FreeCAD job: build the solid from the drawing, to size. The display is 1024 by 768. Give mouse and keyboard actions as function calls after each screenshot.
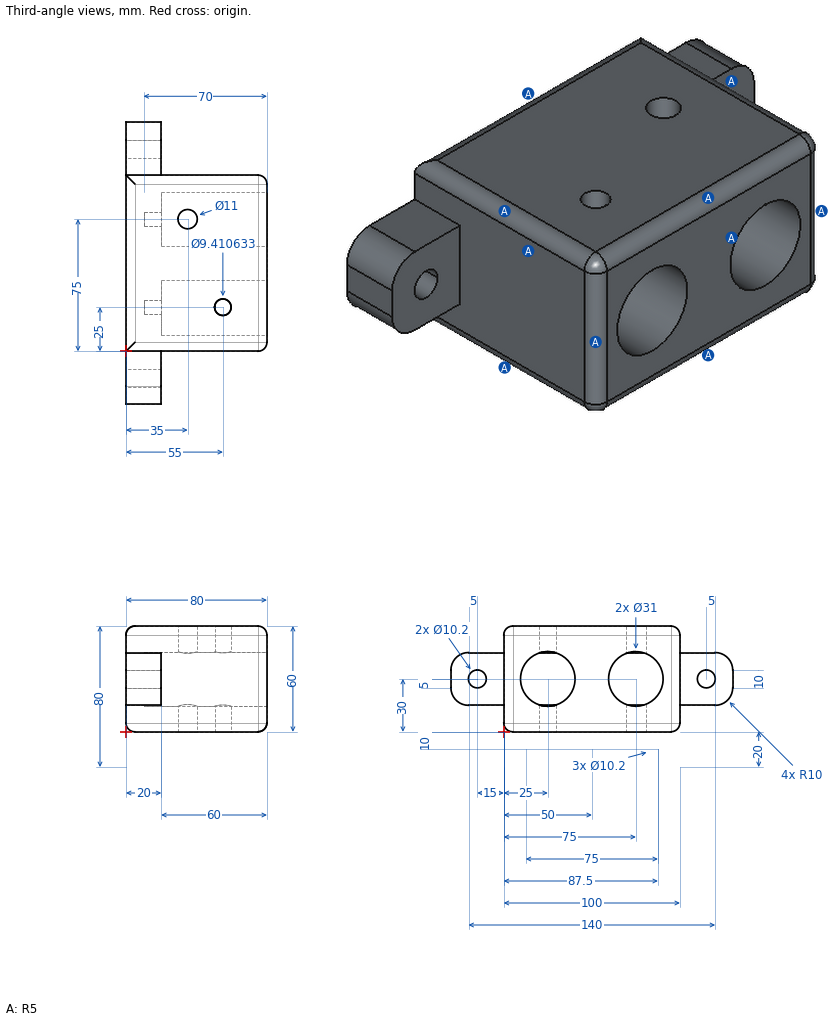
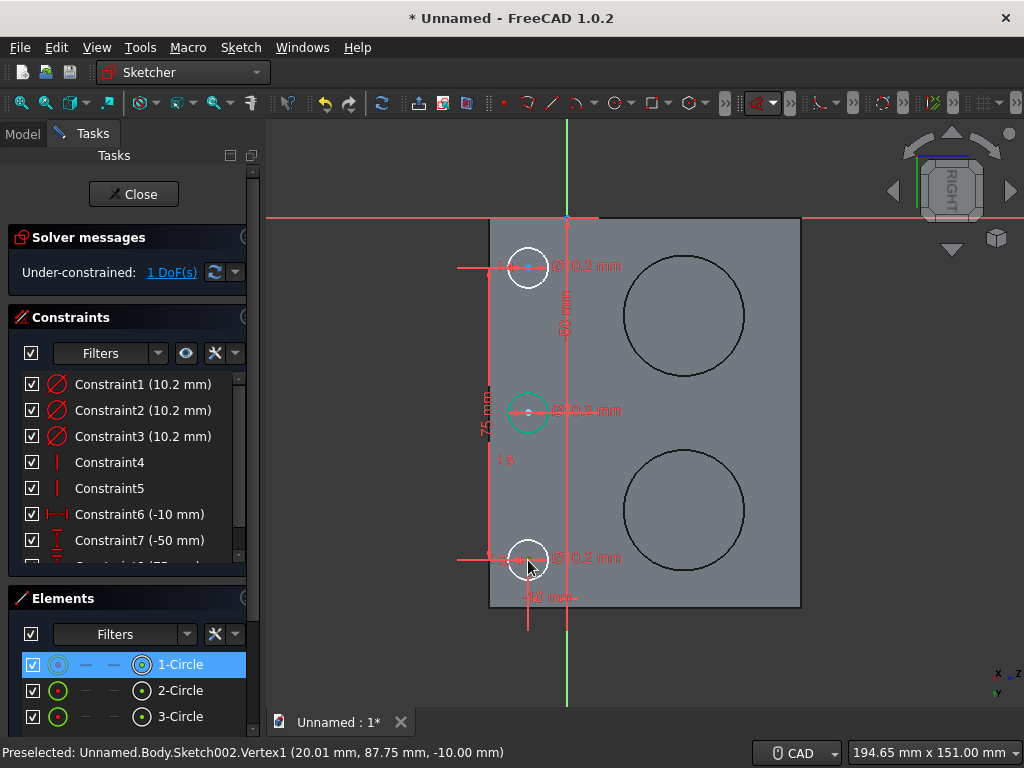
key(i)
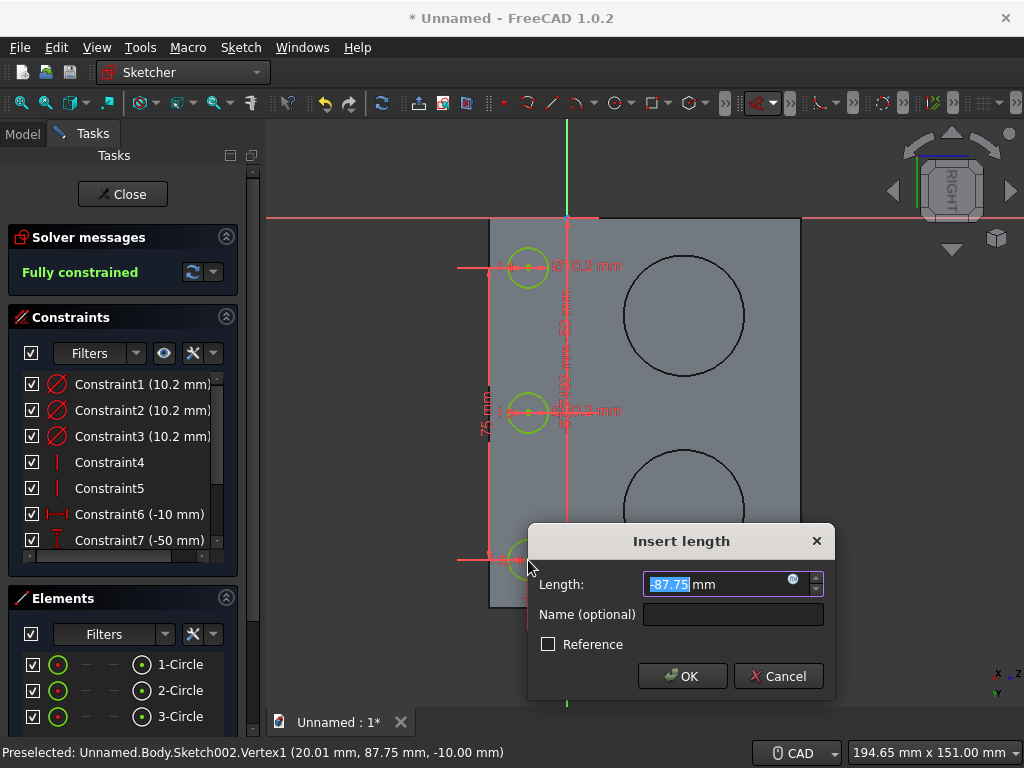
text(-87.5)
key(Return)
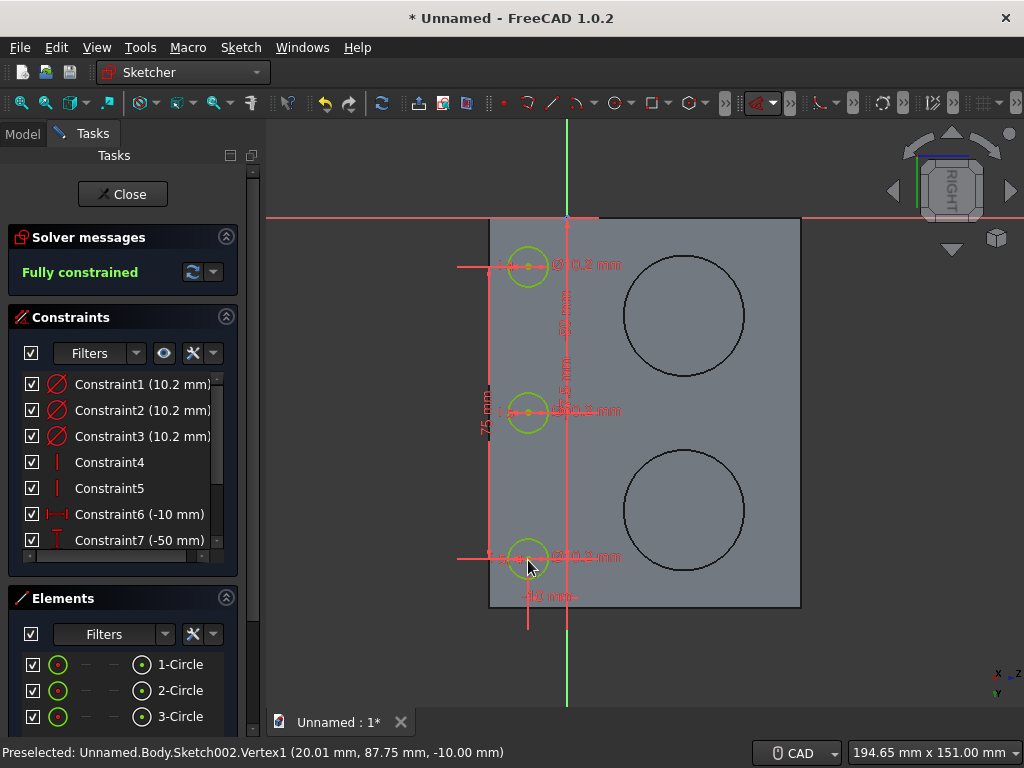
click(123, 194)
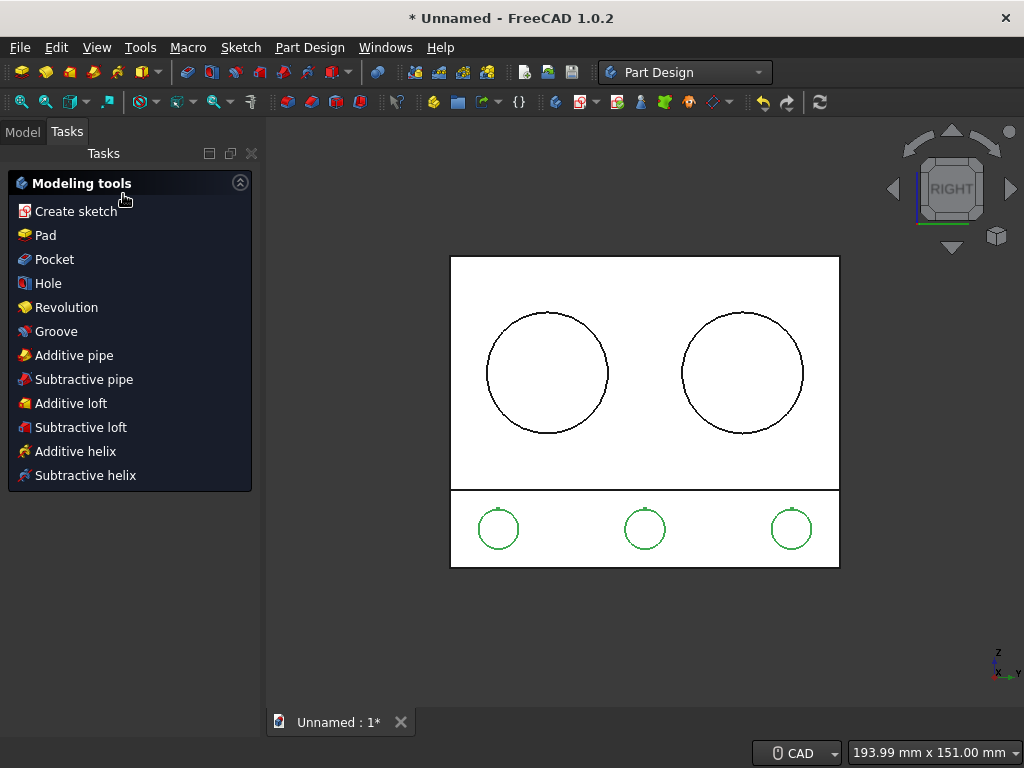
click(188, 72)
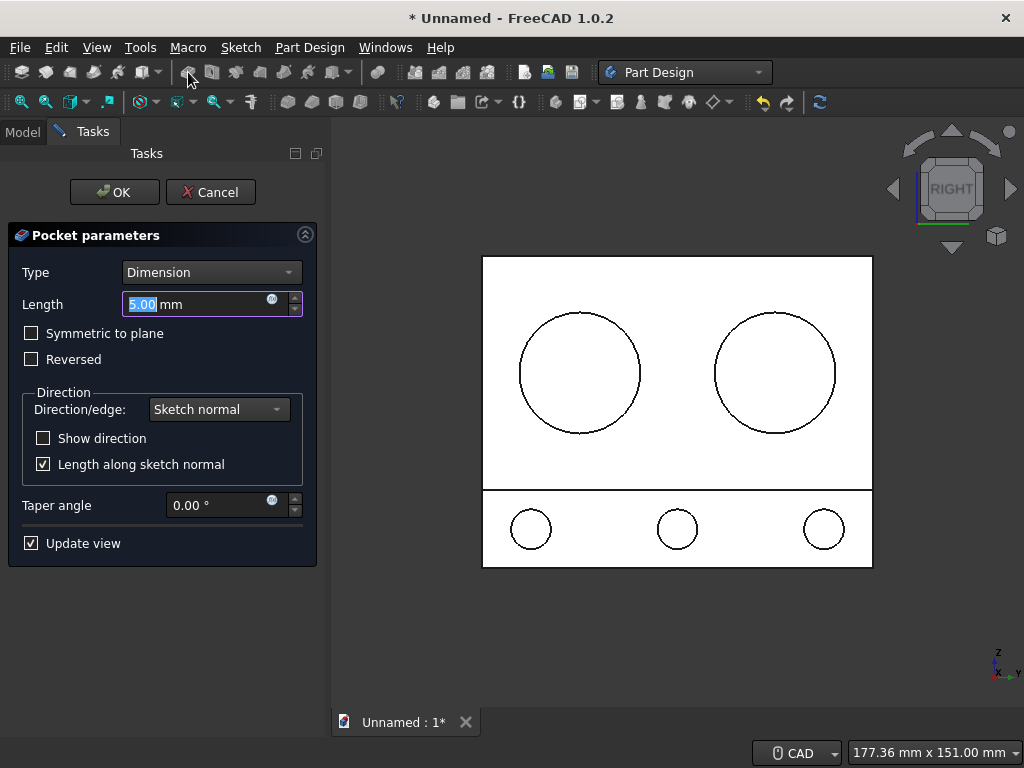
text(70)
key(Tab)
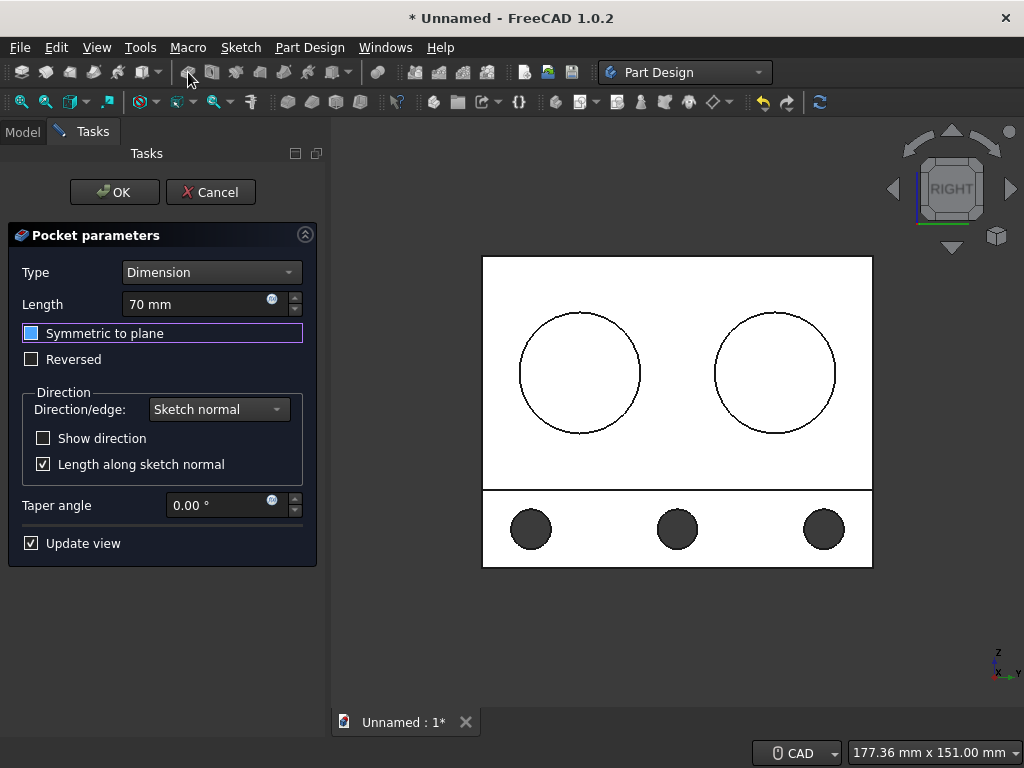
click(115, 192)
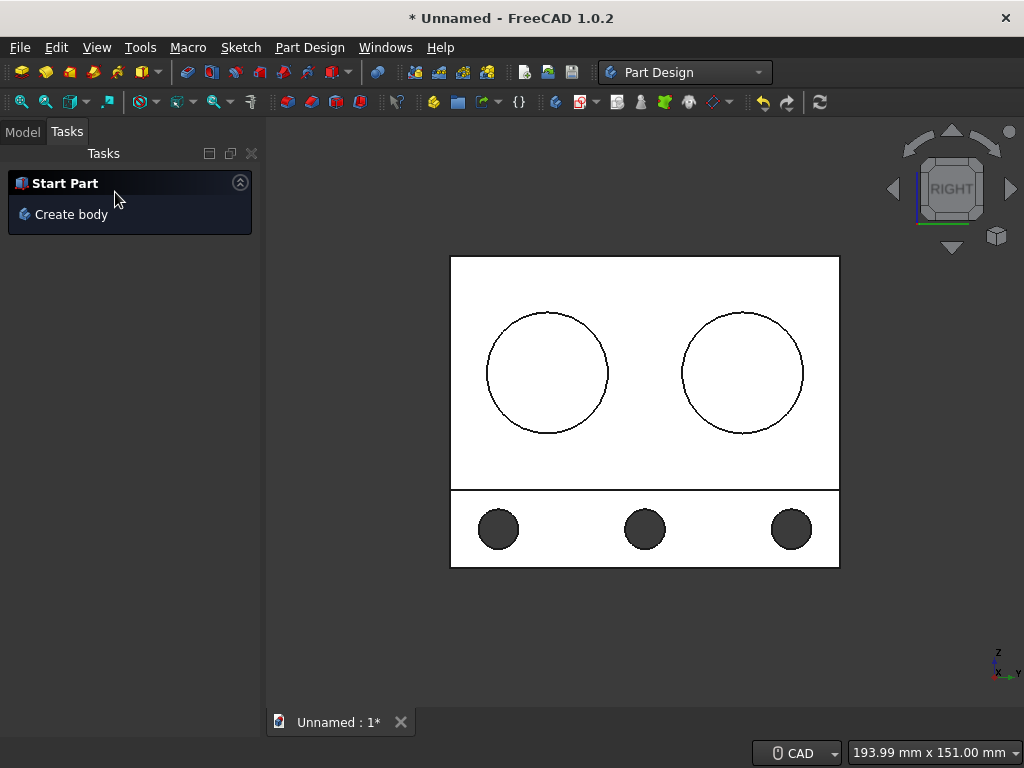
key(5)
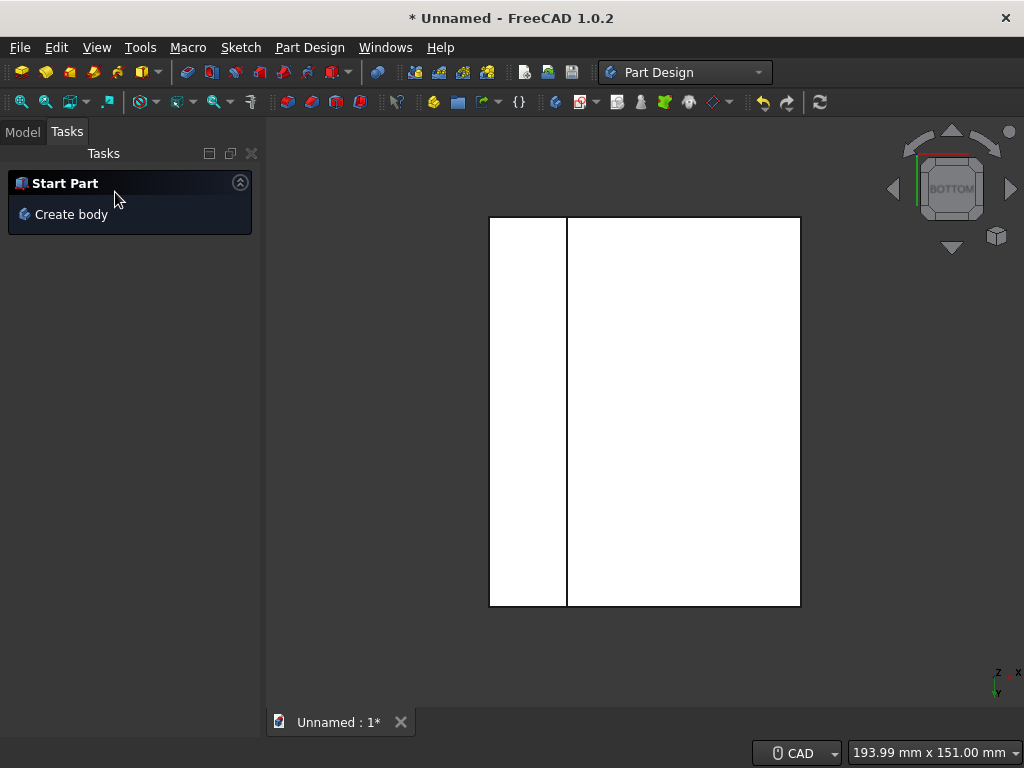
click(684, 467)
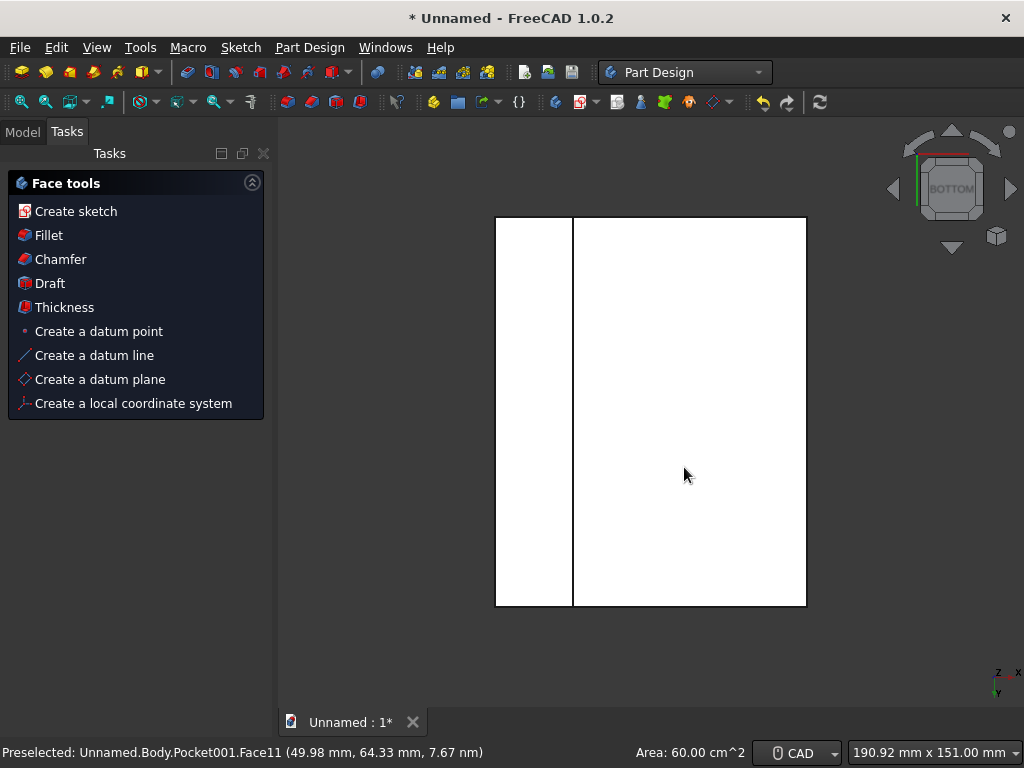
click(580, 102)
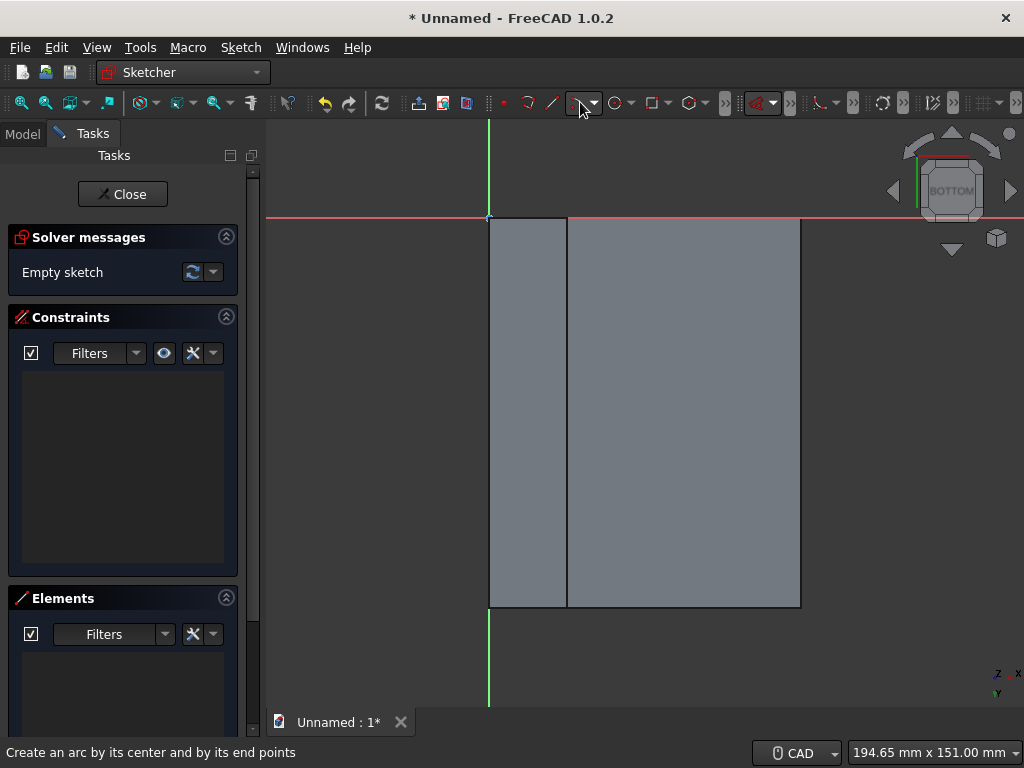
key(q)
key(s)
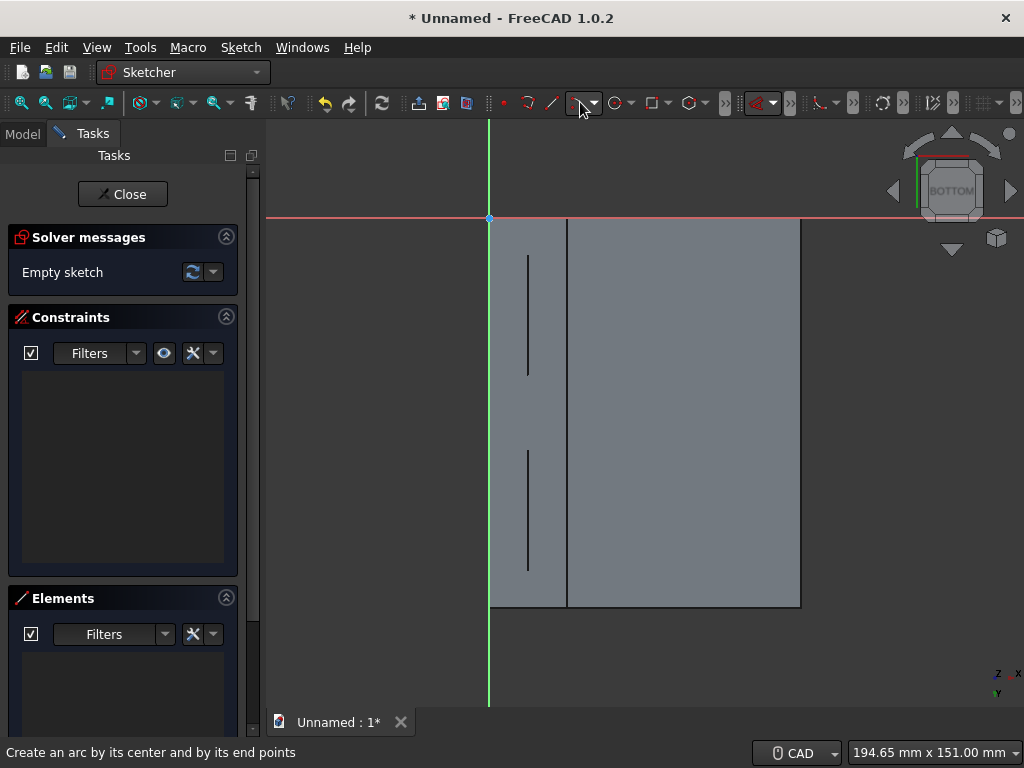
click(616, 104)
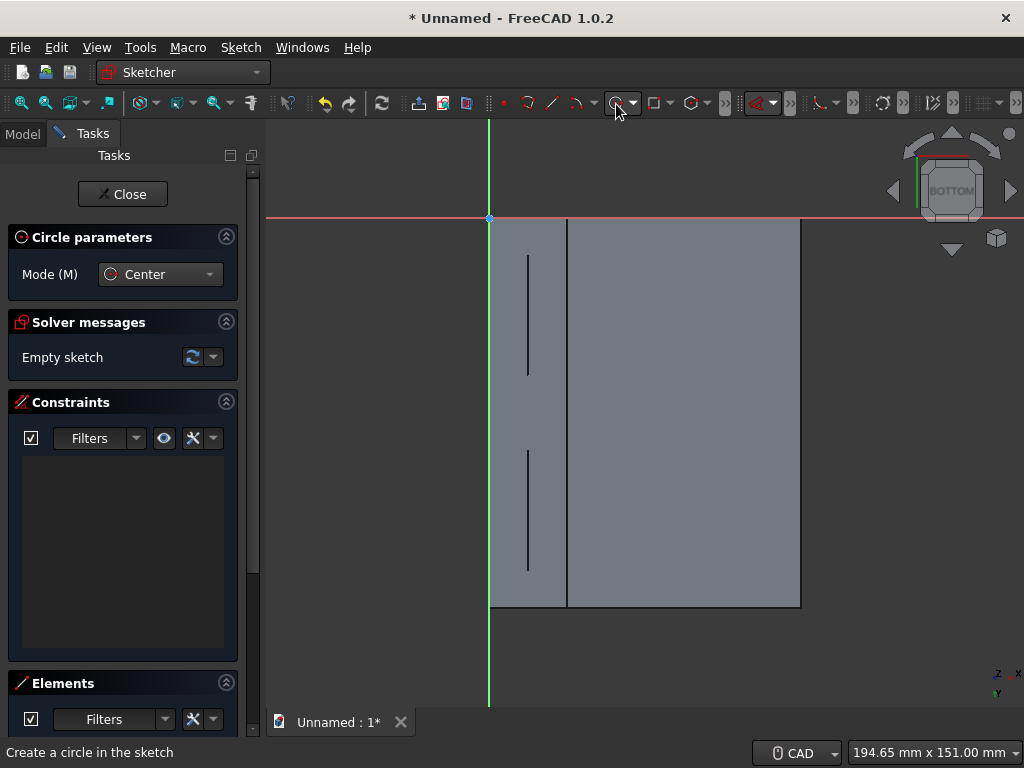
click(626, 510)
move(641, 495)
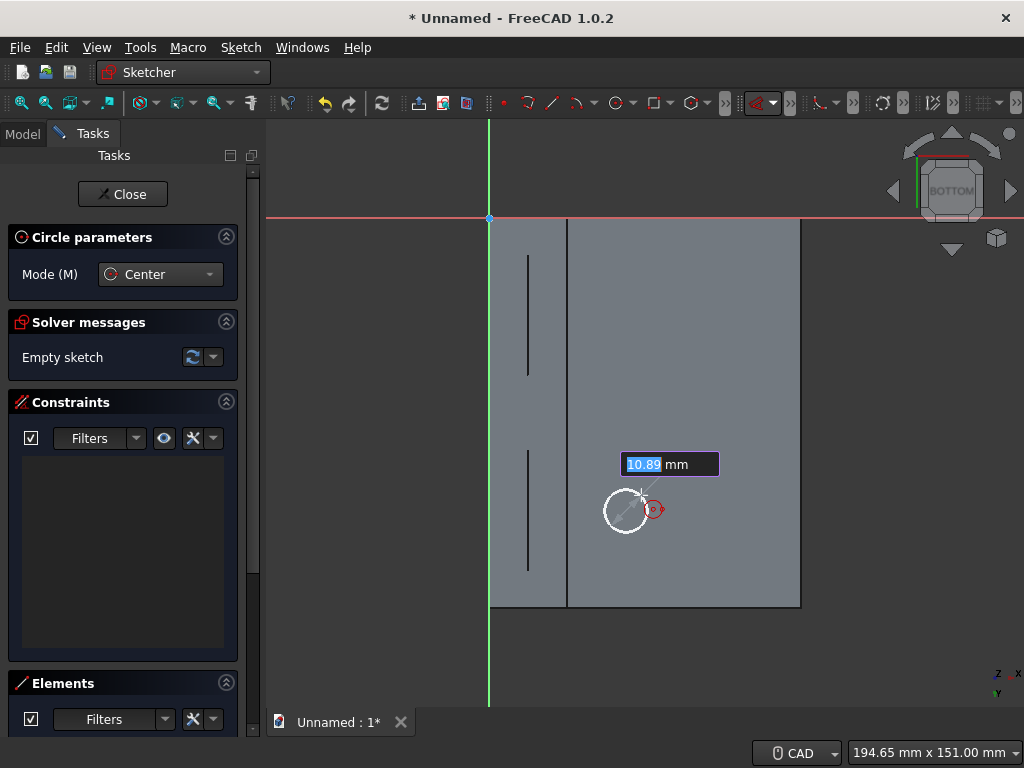
text(11)
key(Return)